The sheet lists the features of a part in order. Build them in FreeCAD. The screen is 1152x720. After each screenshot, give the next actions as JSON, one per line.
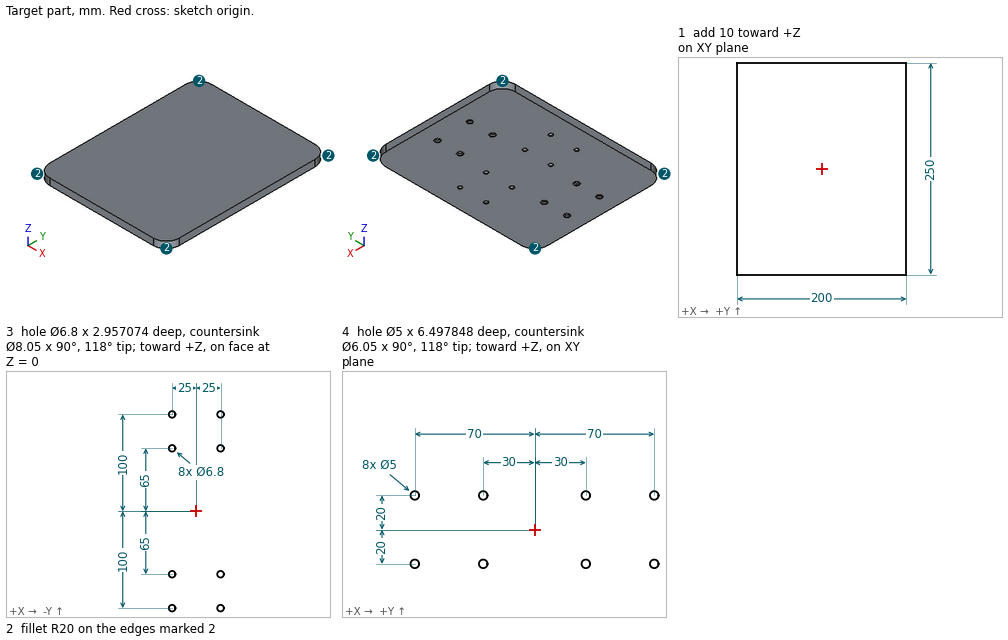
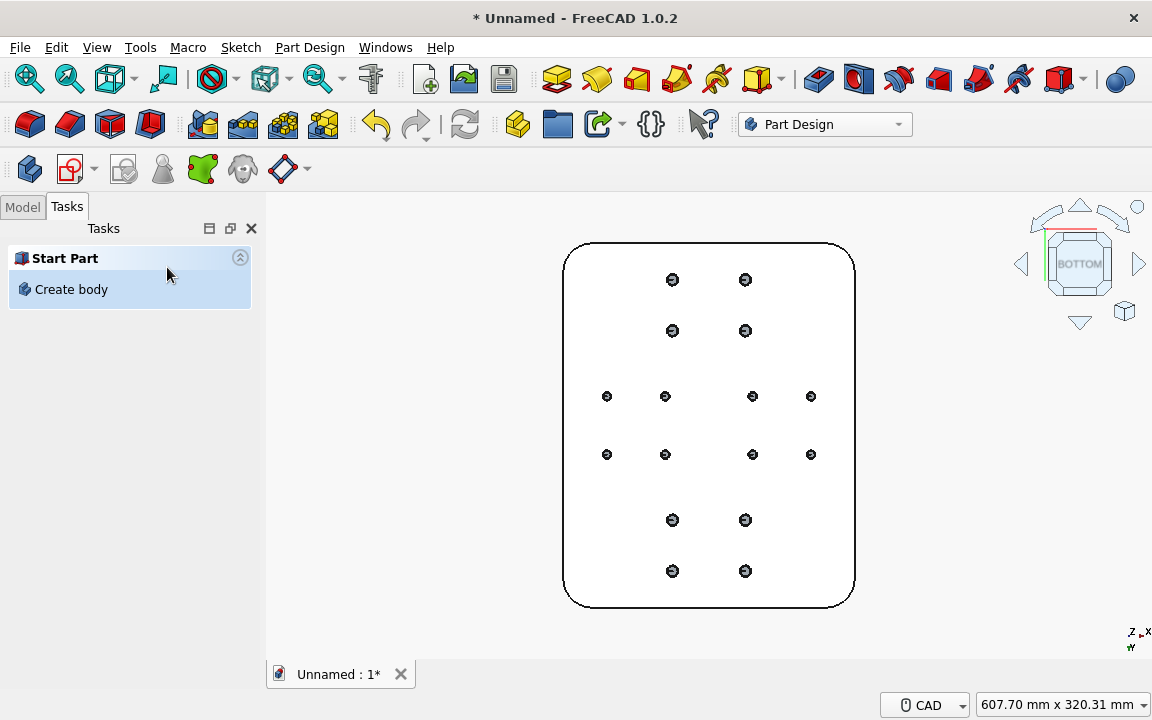
{"action": "key", "text": "0"}